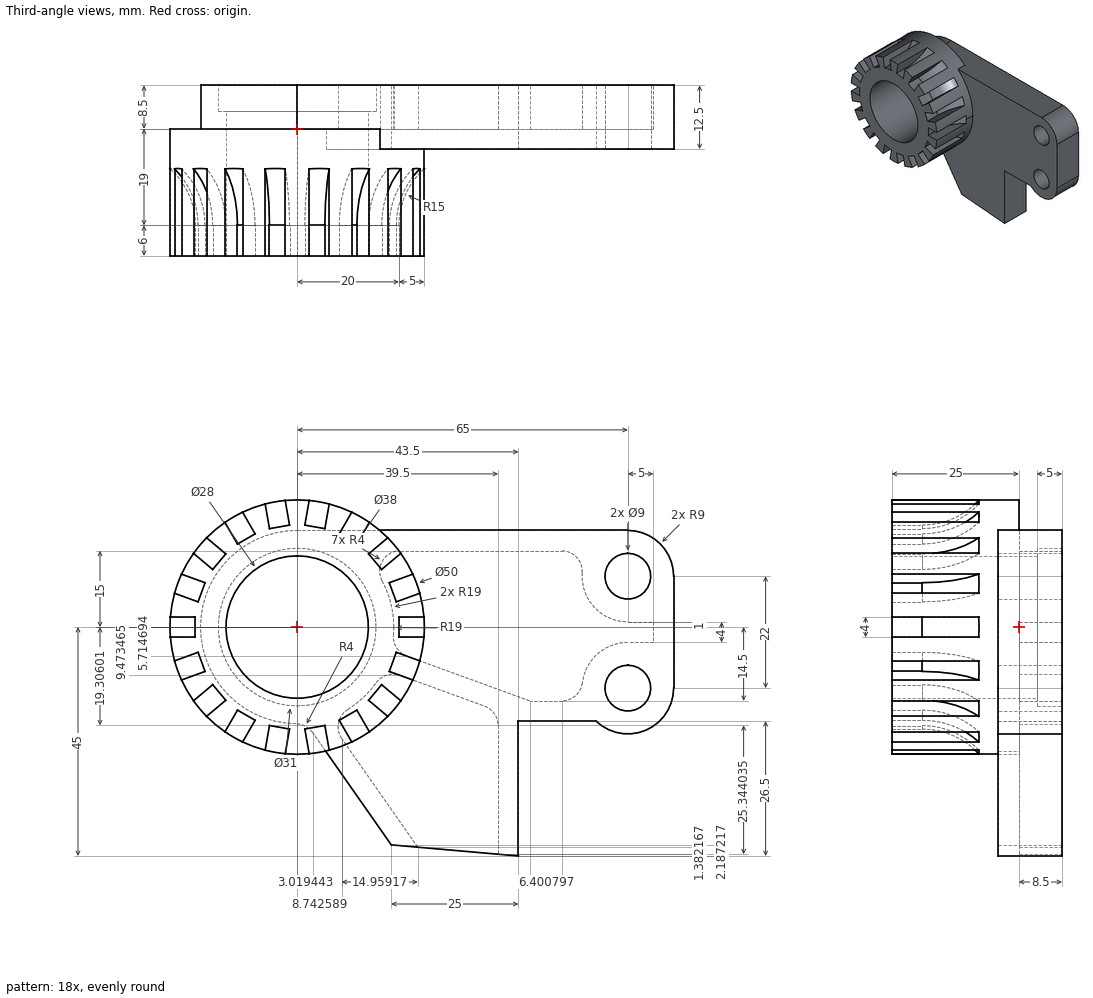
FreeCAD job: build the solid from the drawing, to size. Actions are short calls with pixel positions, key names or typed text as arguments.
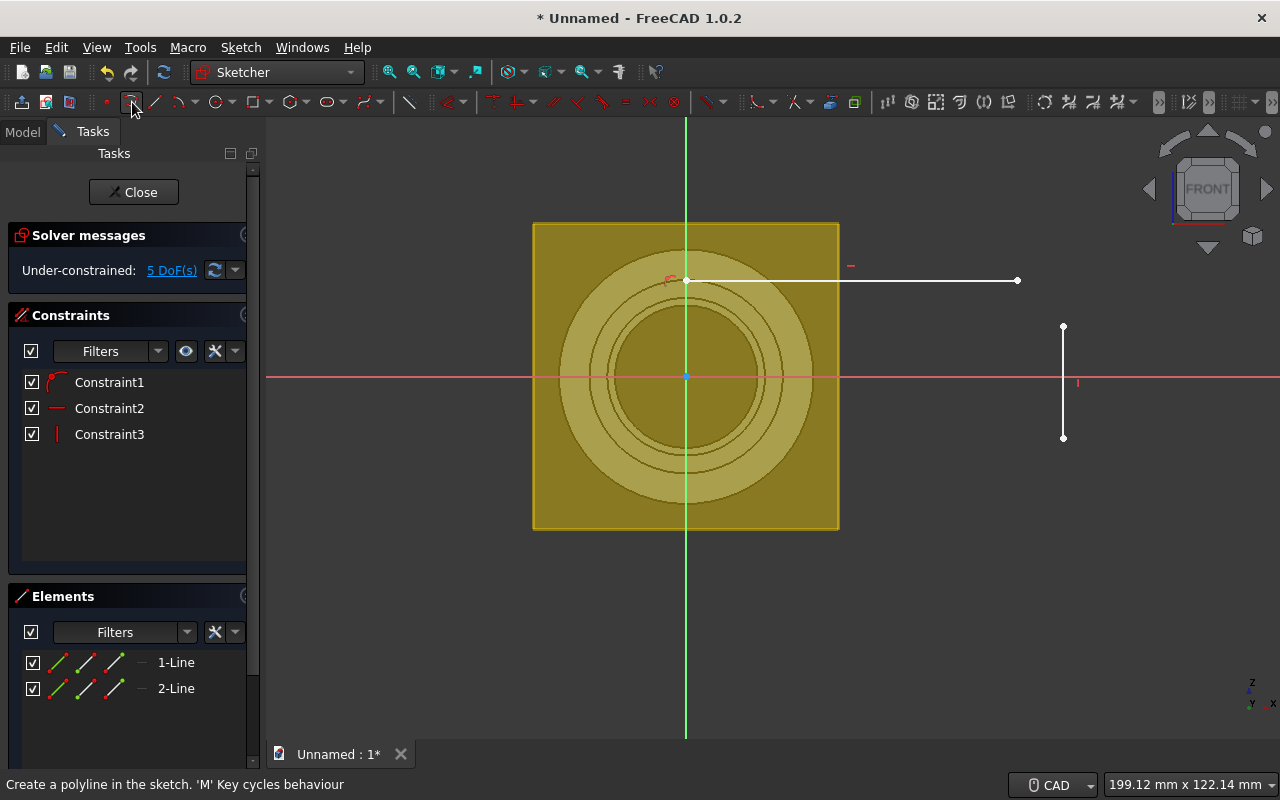
click(985, 471)
click(908, 471)
click(908, 606)
click(780, 595)
click(702, 482)
right_click(702, 482)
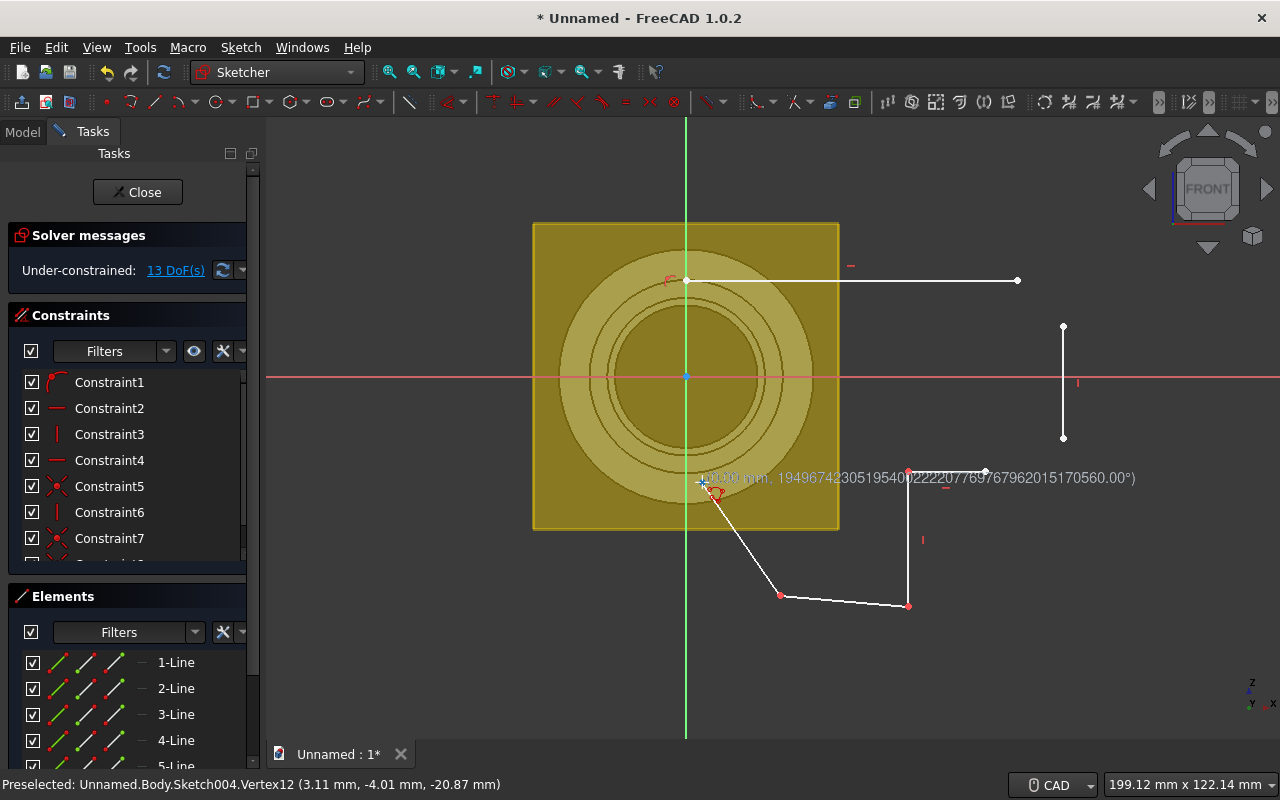
click(198, 102)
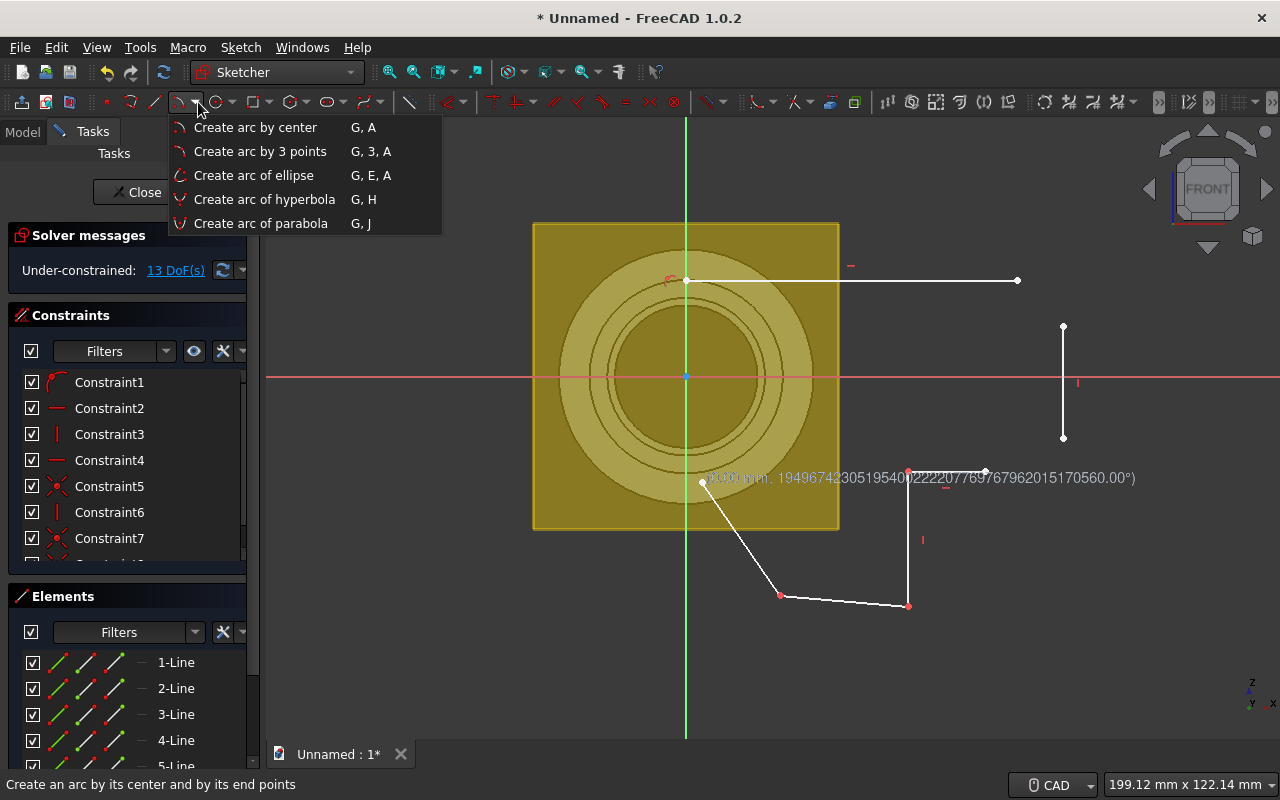
click(306, 151)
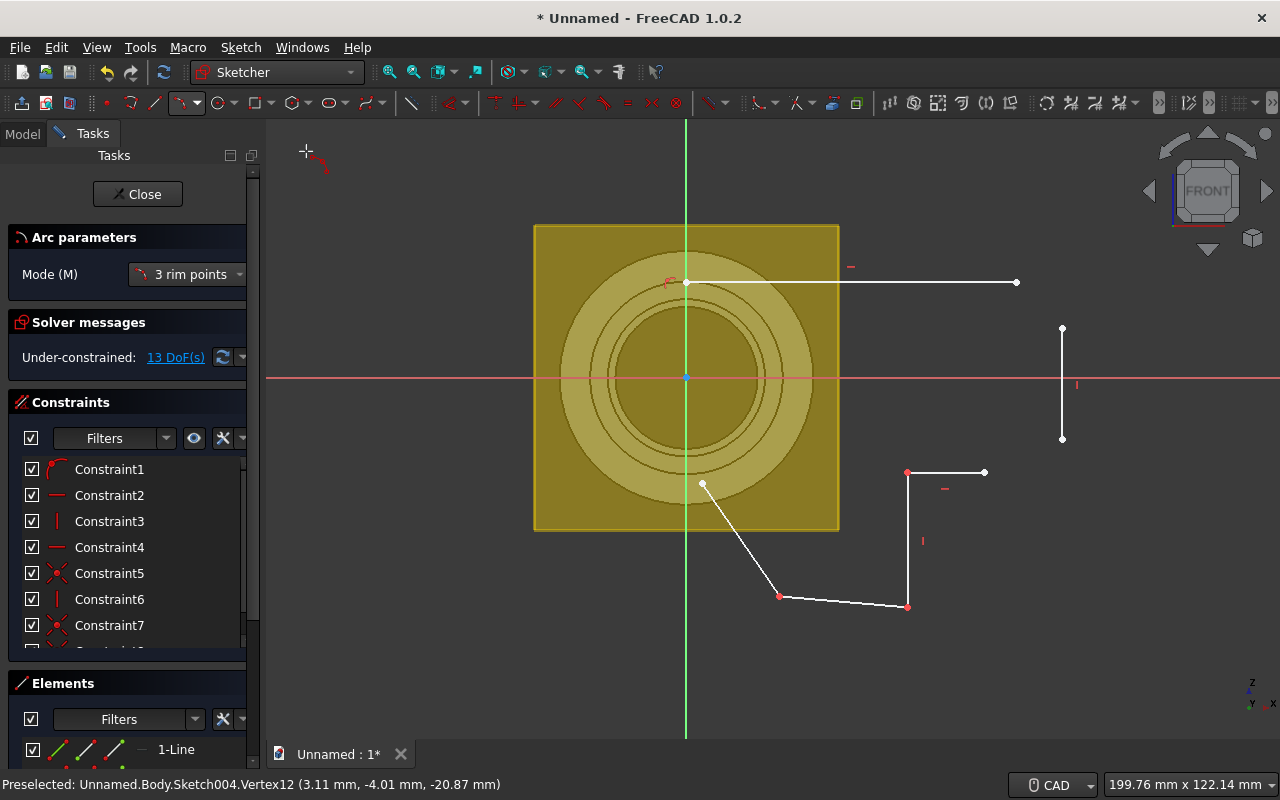
click(1016, 282)
click(1062, 328)
click(1049, 295)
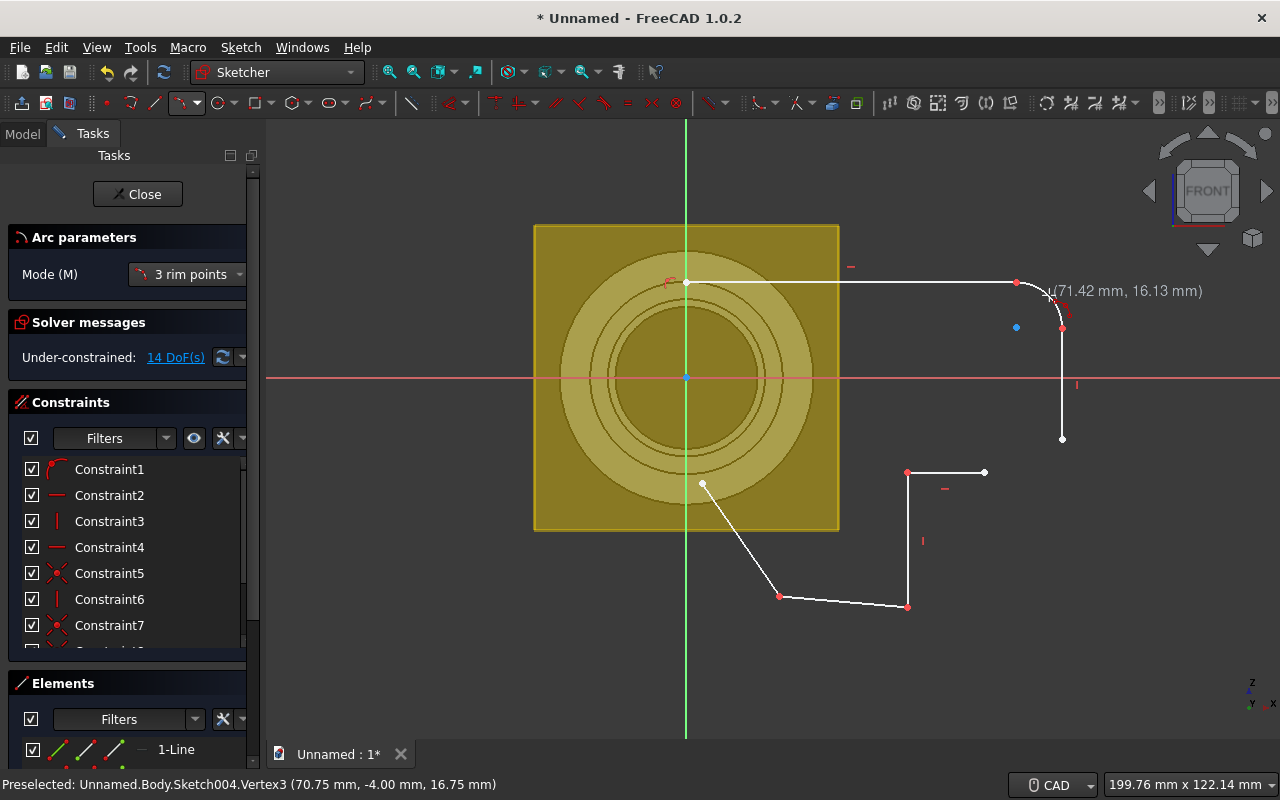
click(1062, 440)
click(984, 473)
click(1034, 481)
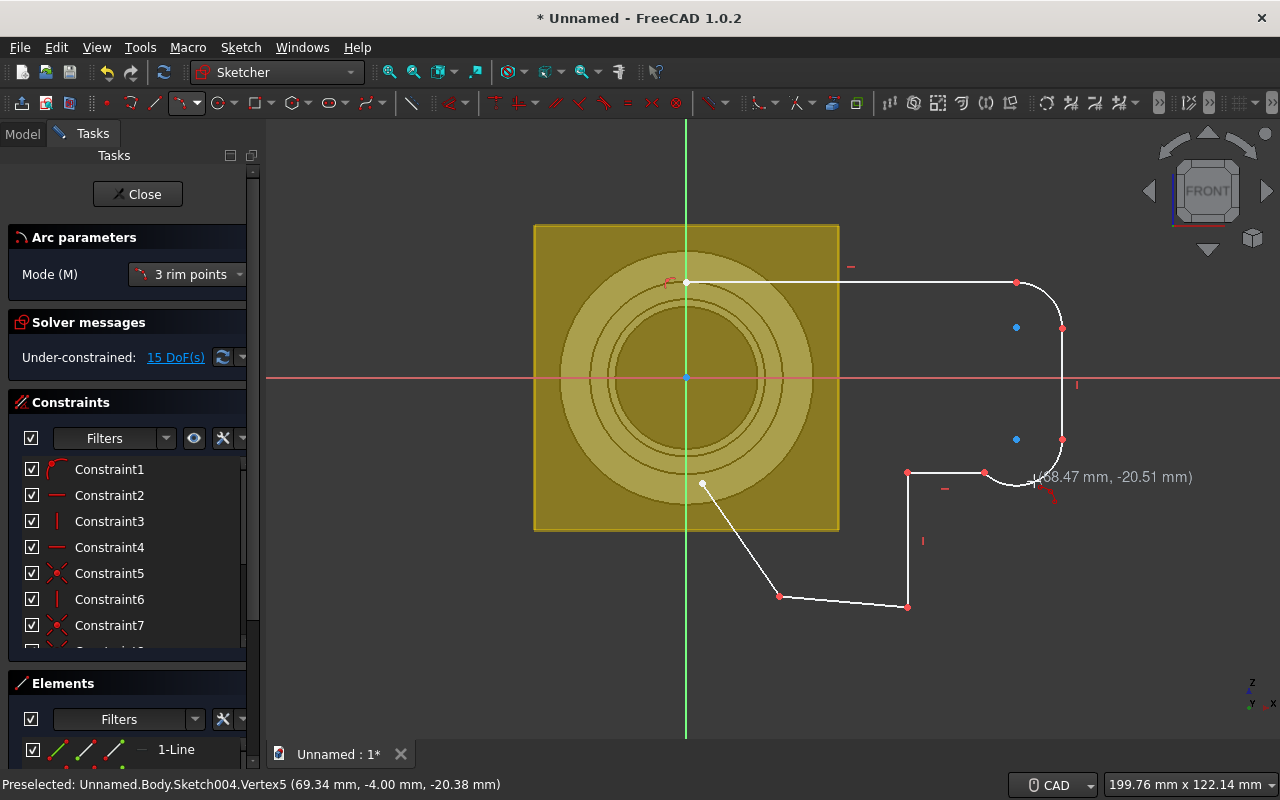
click(702, 484)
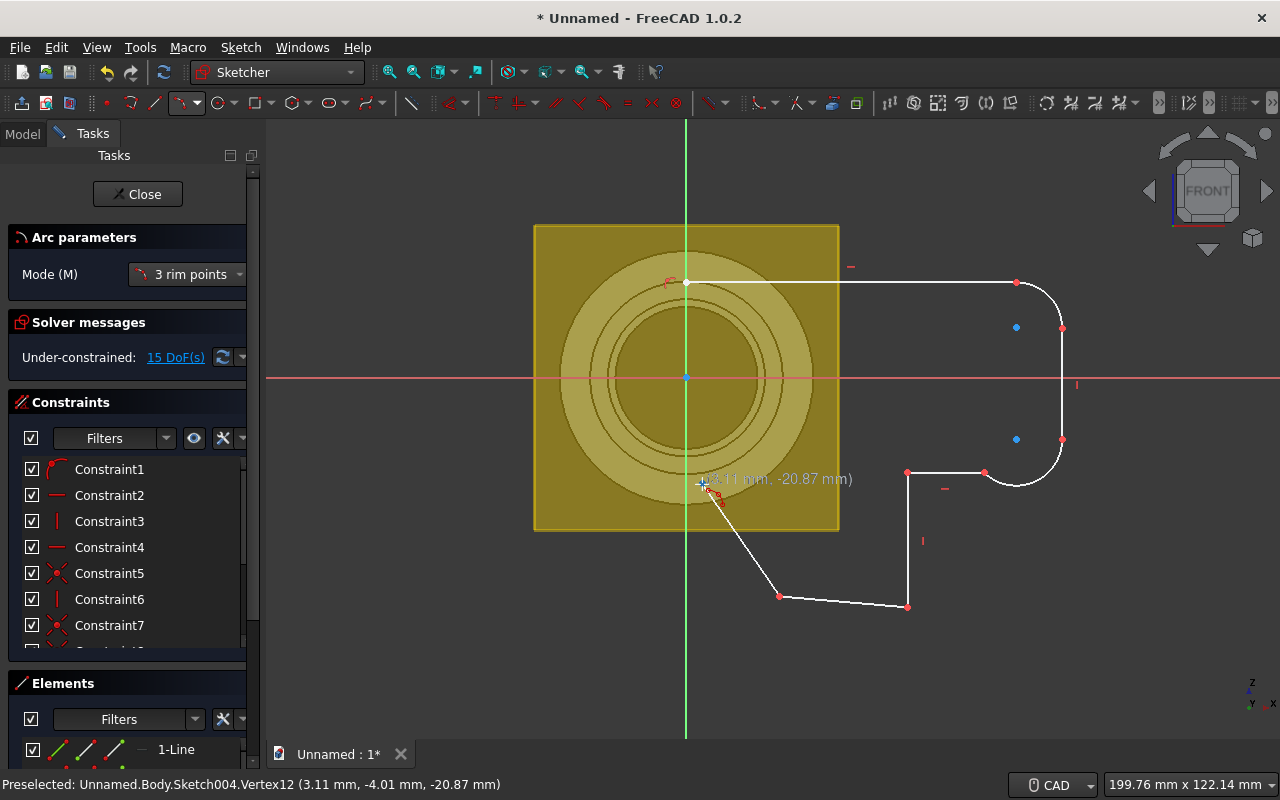
scroll(685, 474, up, 14)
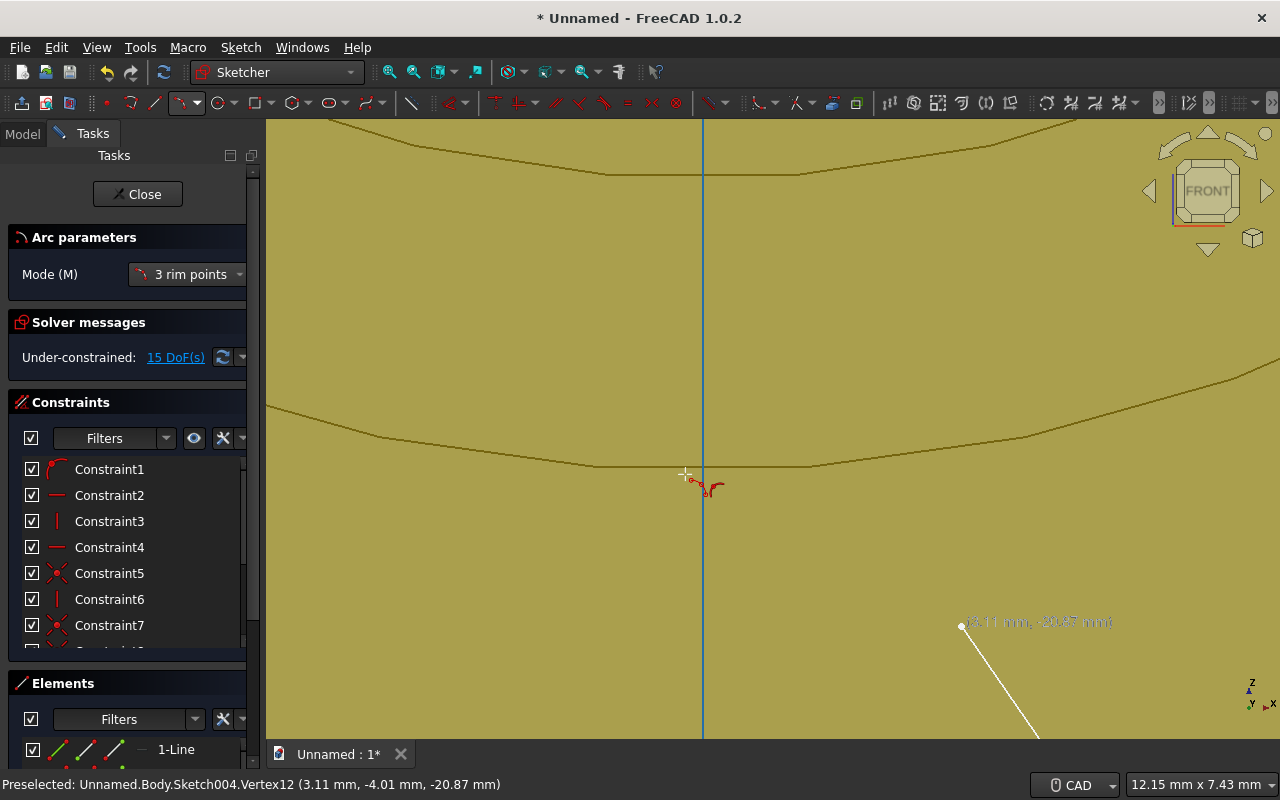
click(685, 470)
click(837, 509)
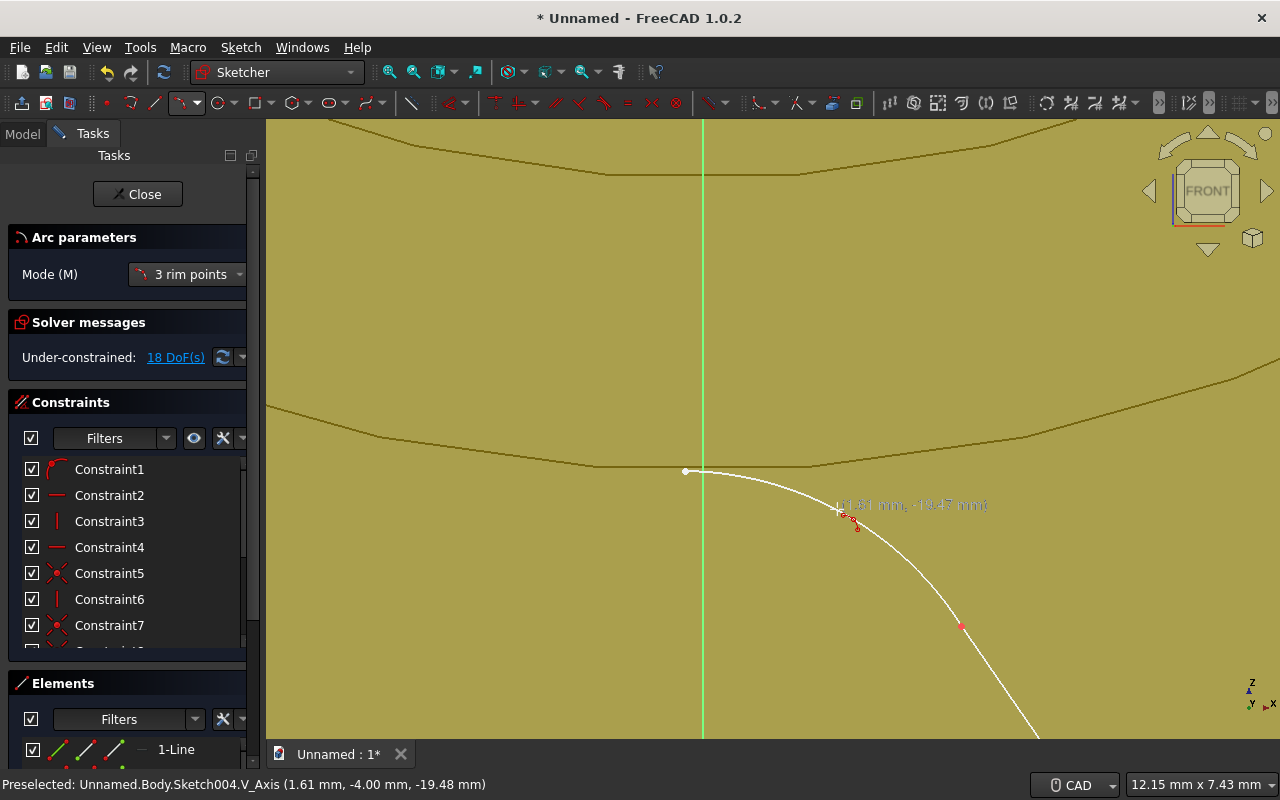
click(685, 471)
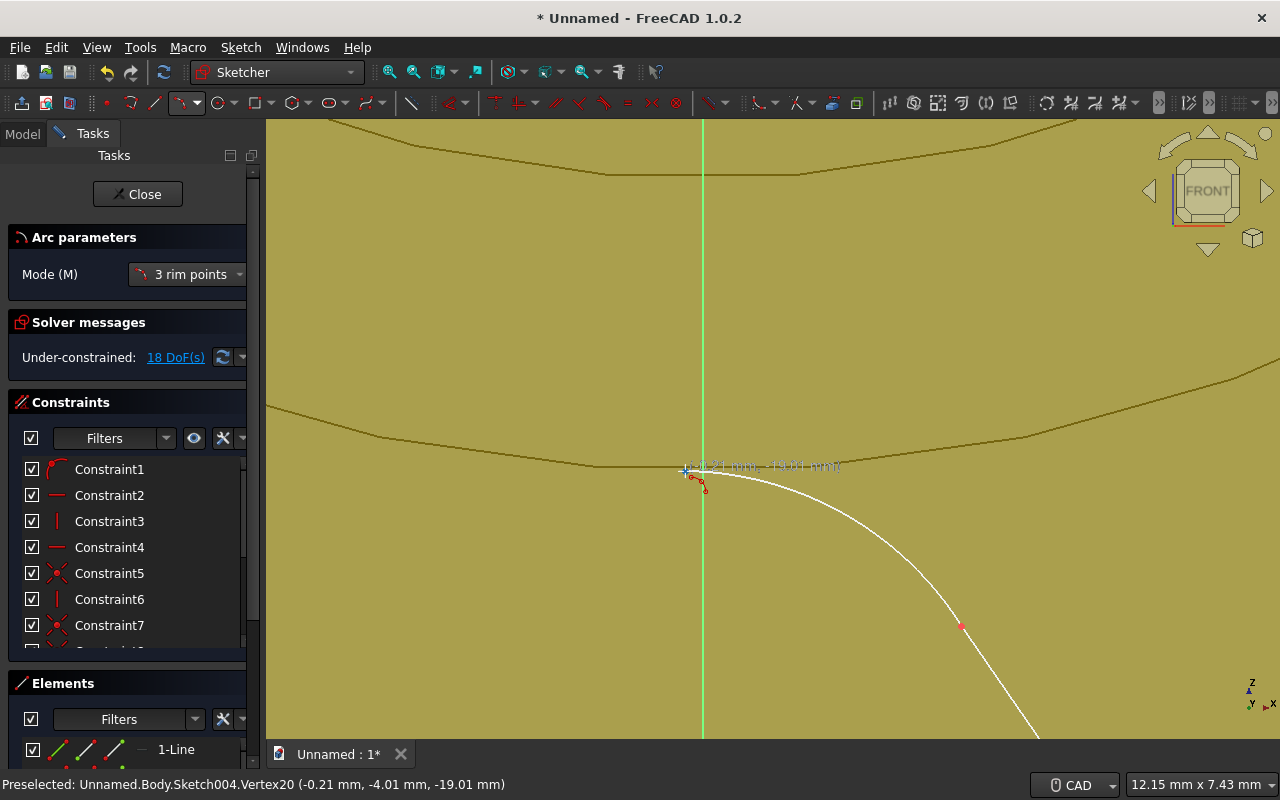
scroll(458, 466, down, 13)